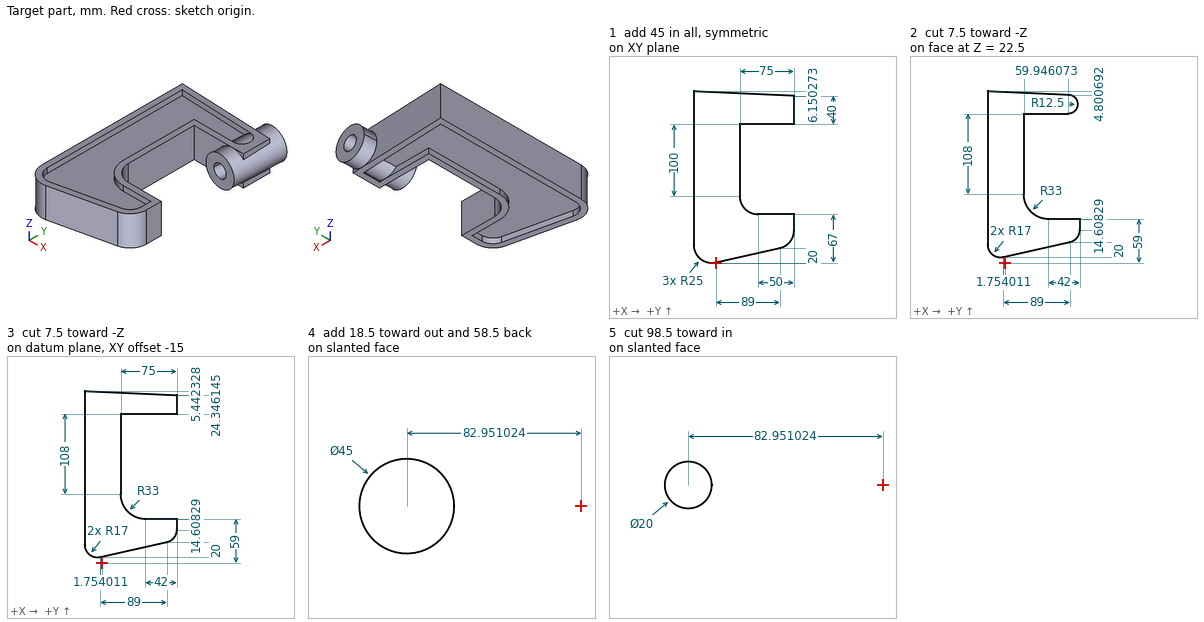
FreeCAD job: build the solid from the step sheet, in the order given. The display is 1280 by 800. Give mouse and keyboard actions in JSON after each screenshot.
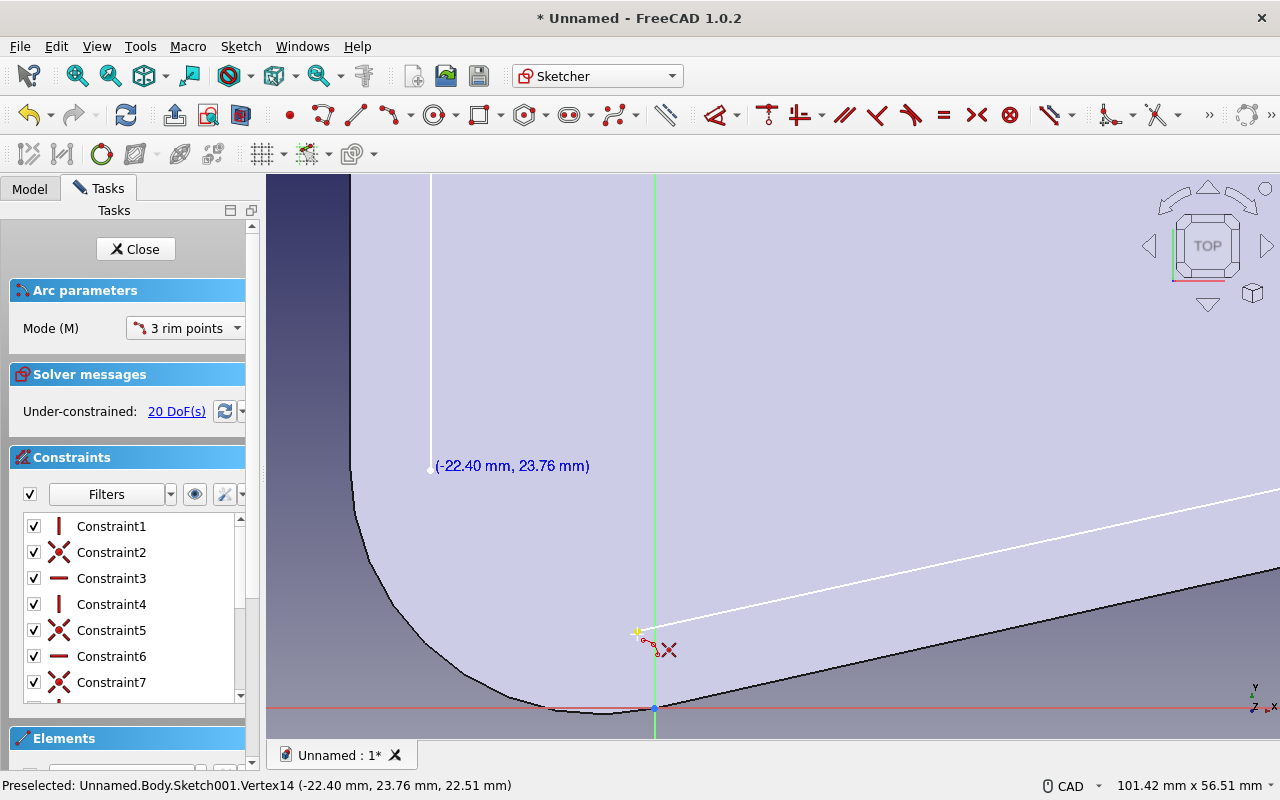
{"action": "left_click", "coordinate": [637, 631]}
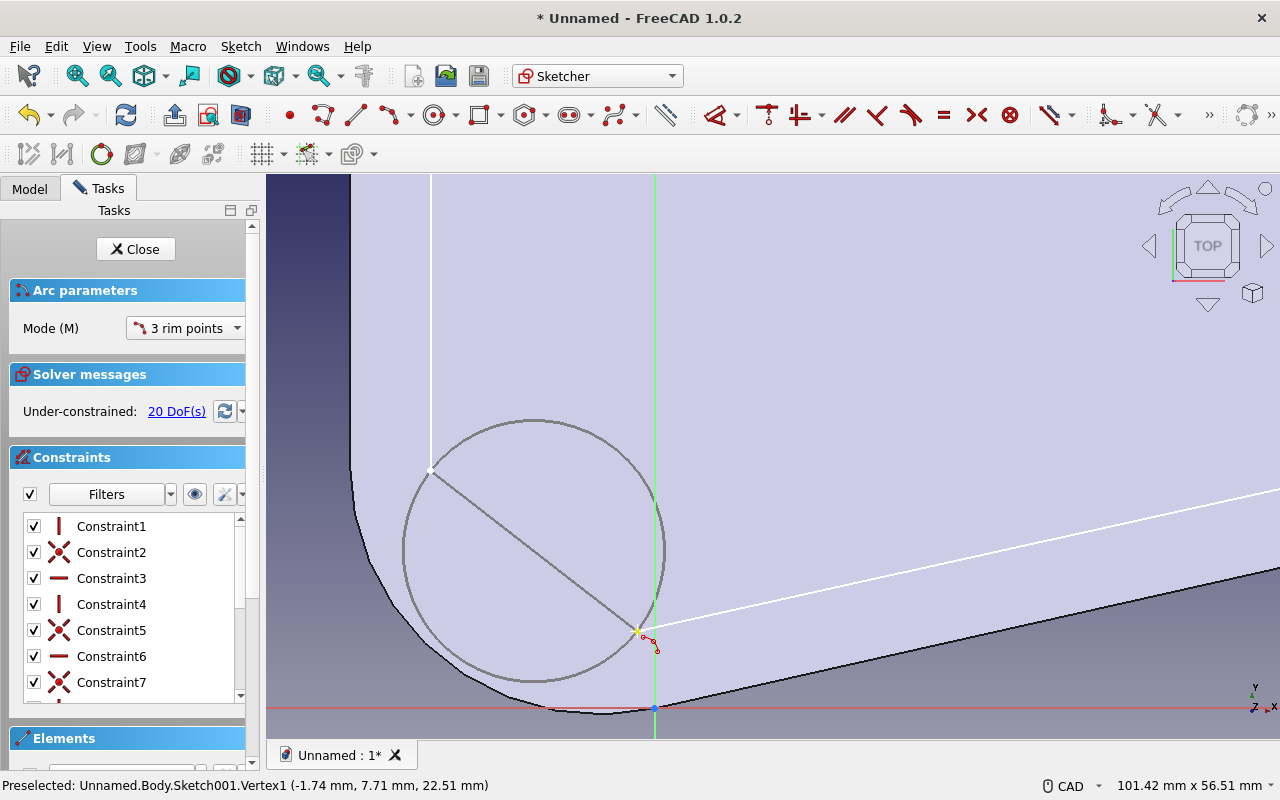
{"action": "scroll", "coordinate": [637, 634], "scroll_direction": "down", "scroll_amount": 9}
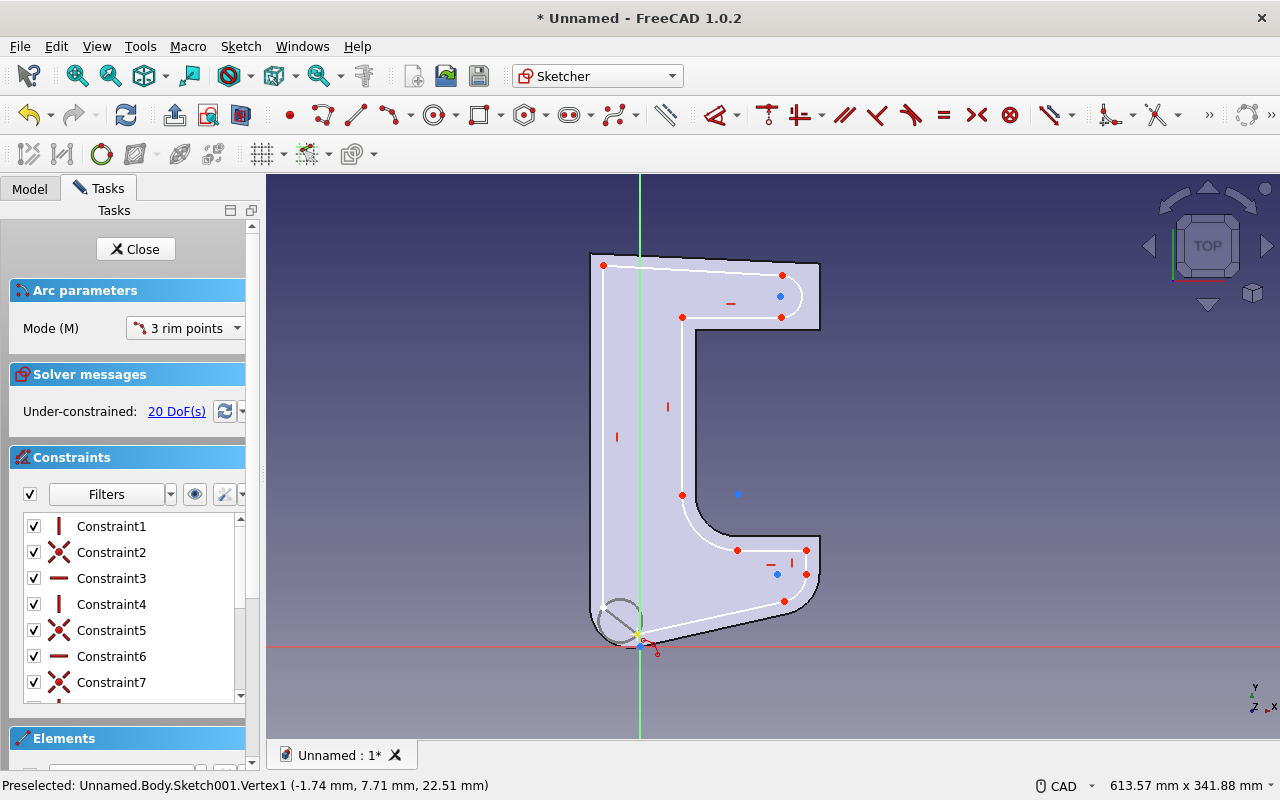
{"action": "scroll", "coordinate": [614, 629], "scroll_direction": "up", "scroll_amount": 3}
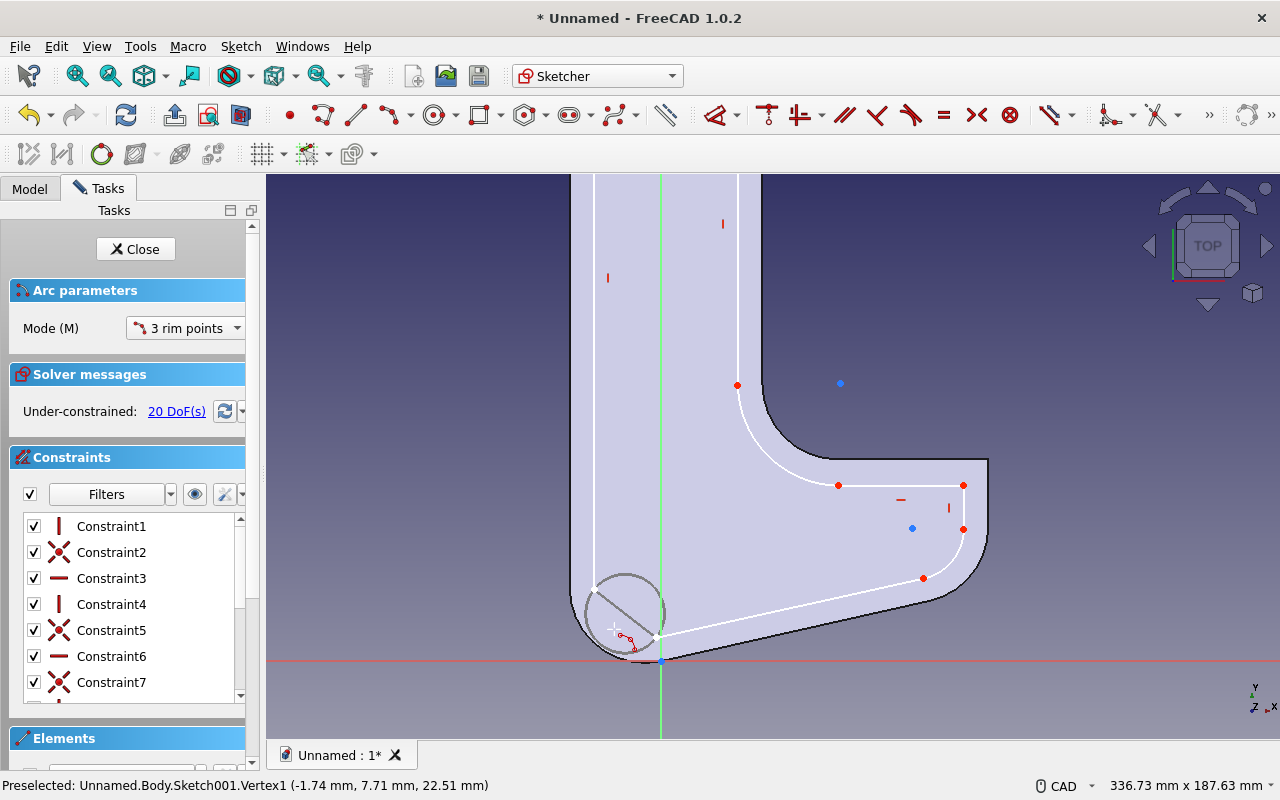
{"action": "left_click", "coordinate": [613, 628]}
{"action": "key", "text": "Escape"}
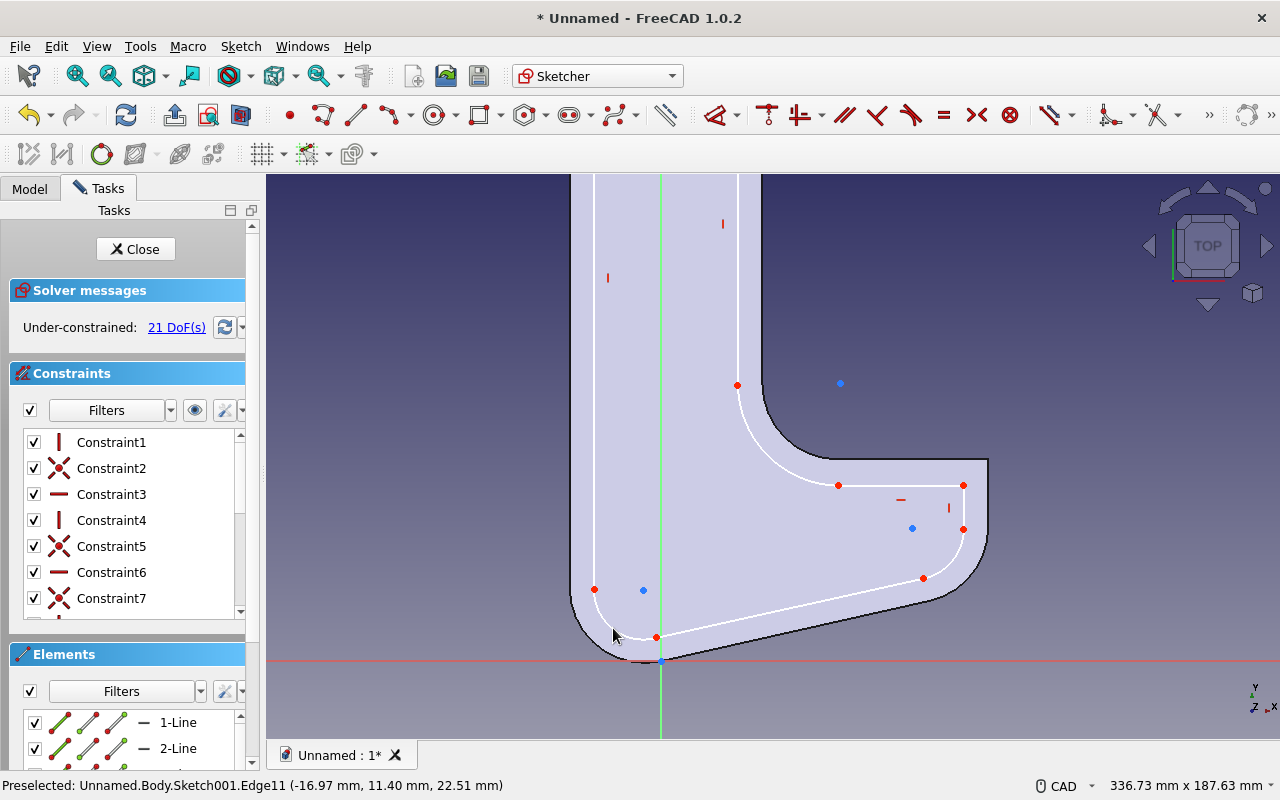
{"action": "left_click", "coordinate": [737, 620]}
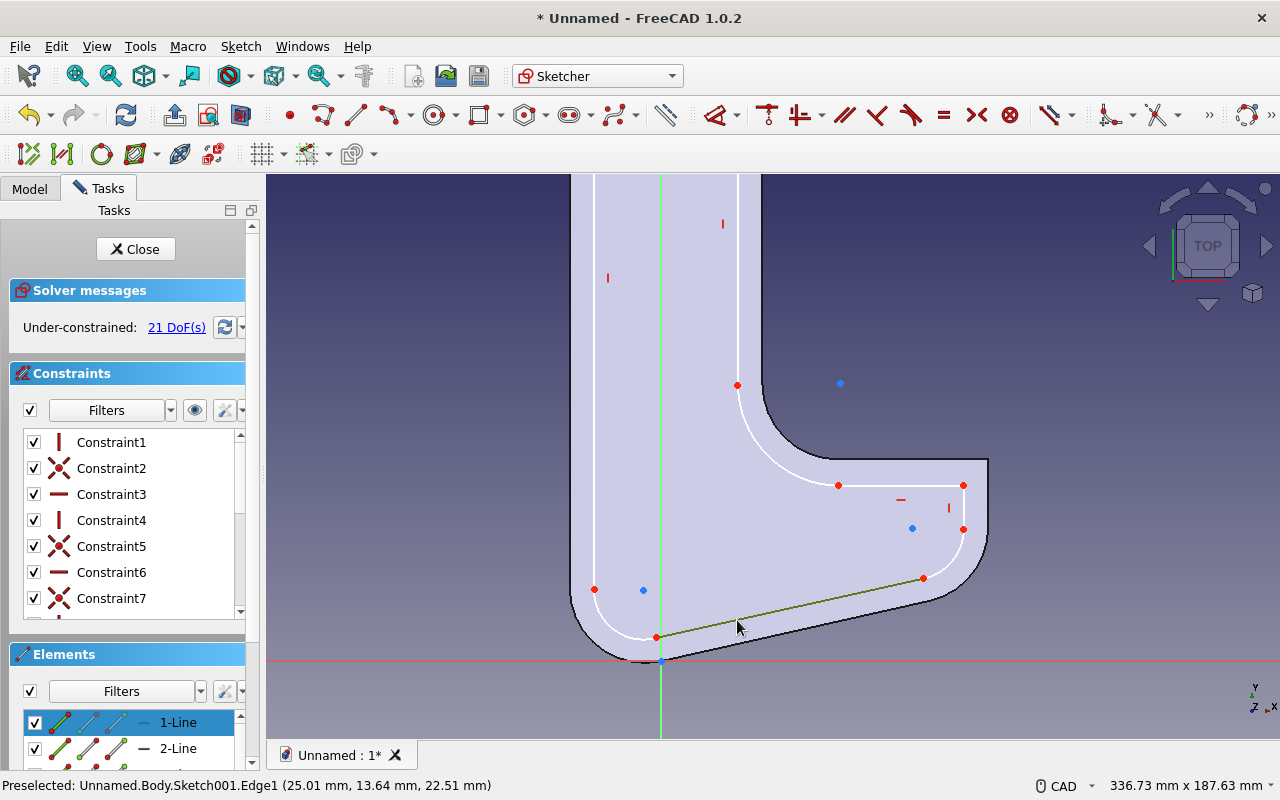
{"action": "left_click", "coordinate": [942, 570]}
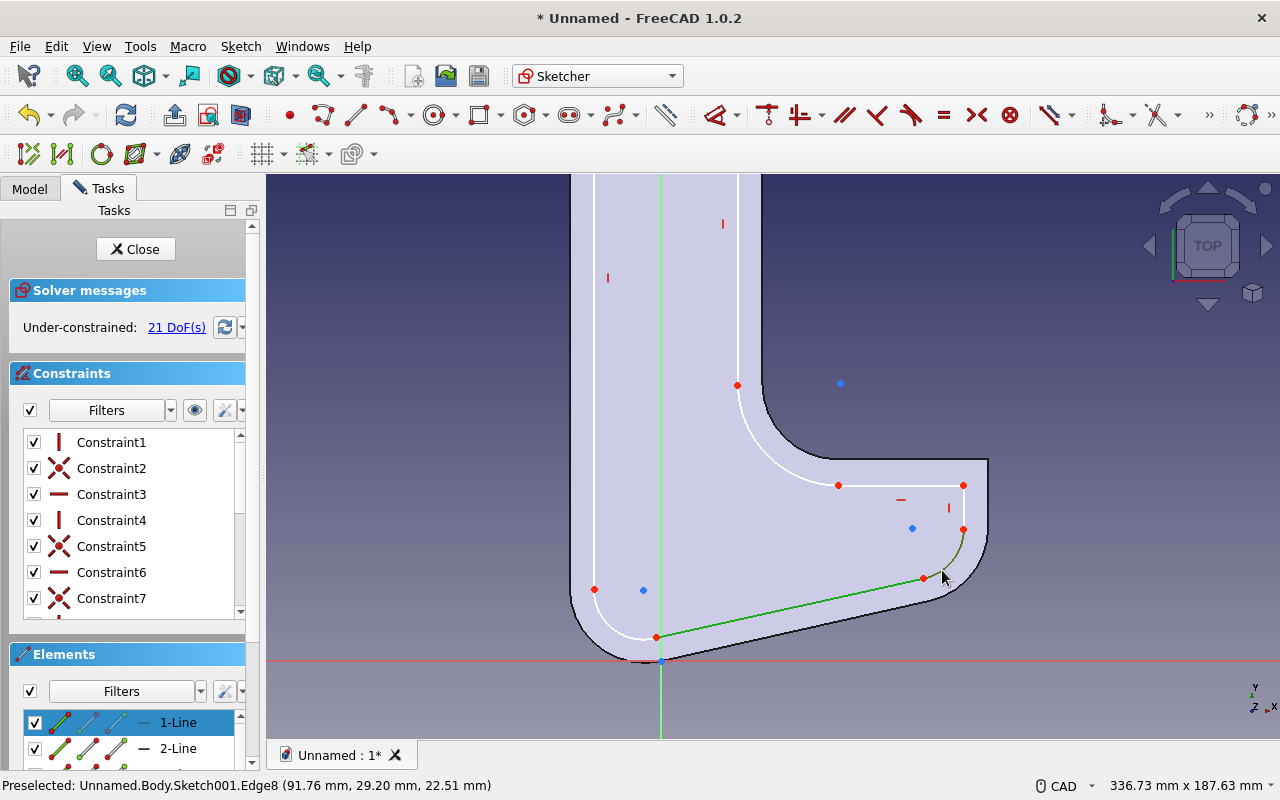
{"action": "key", "text": "t"}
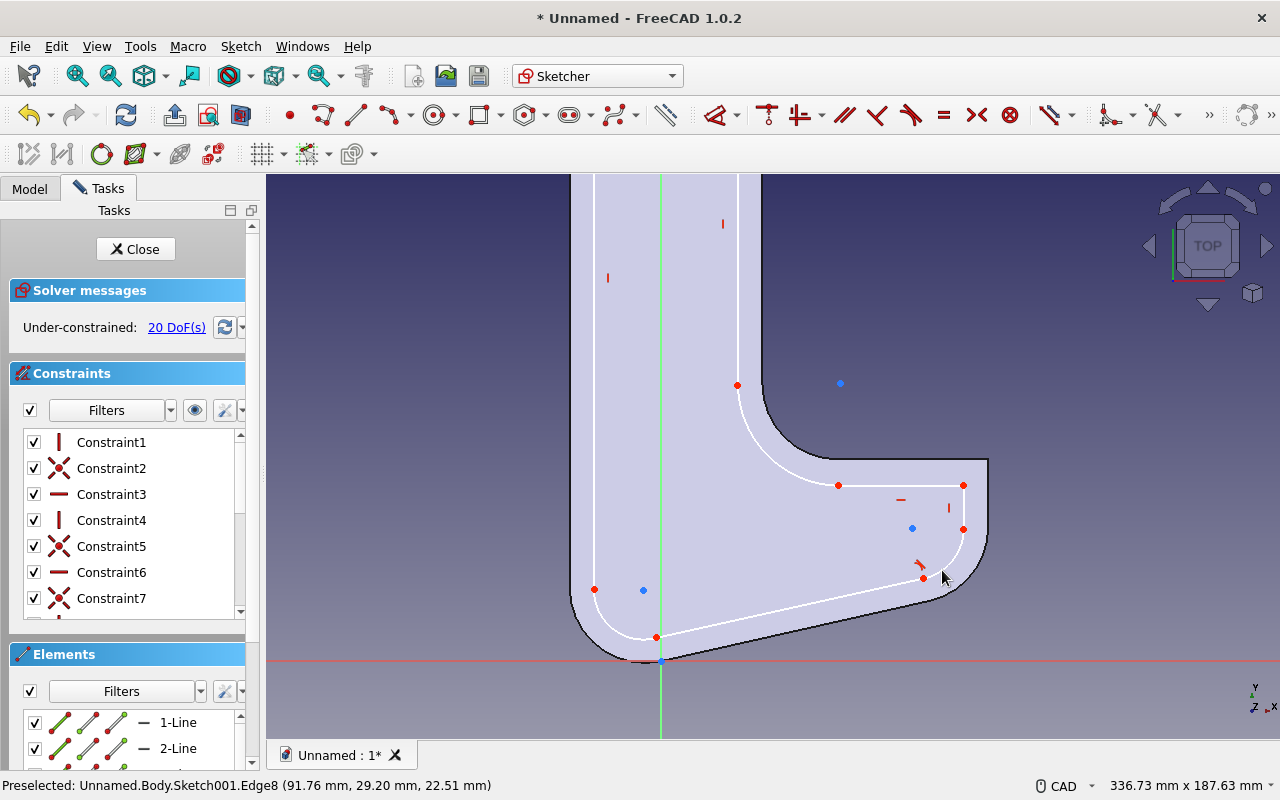
{"action": "left_click", "coordinate": [736, 620]}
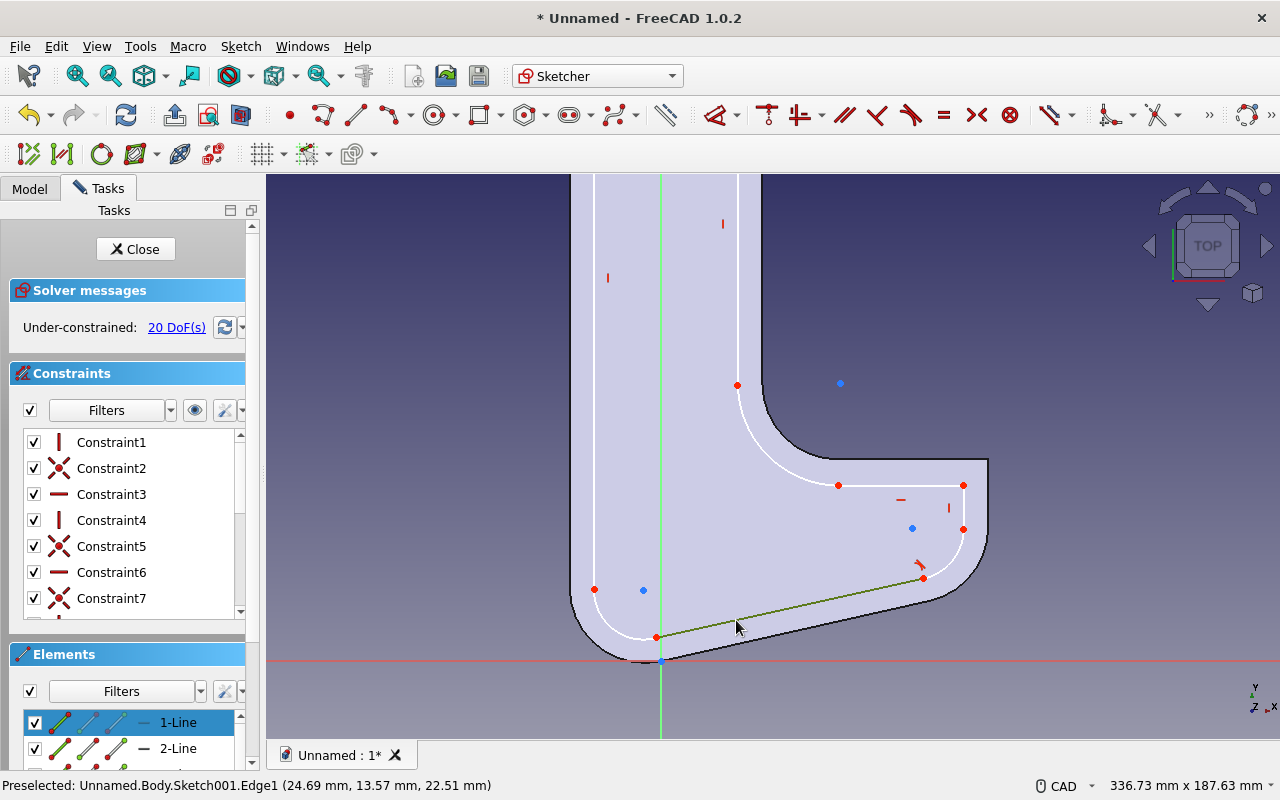
{"action": "left_click", "coordinate": [601, 616]}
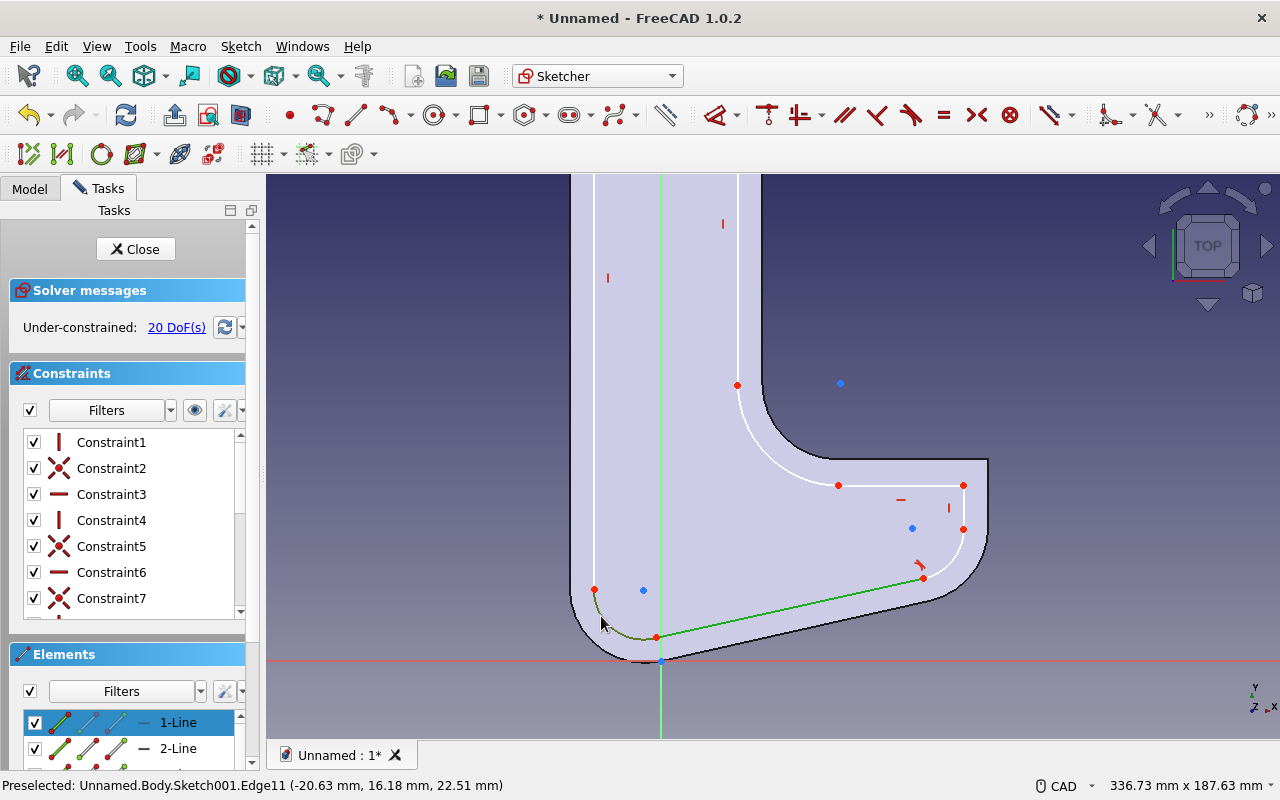
{"action": "left_click", "coordinate": [911, 116]}